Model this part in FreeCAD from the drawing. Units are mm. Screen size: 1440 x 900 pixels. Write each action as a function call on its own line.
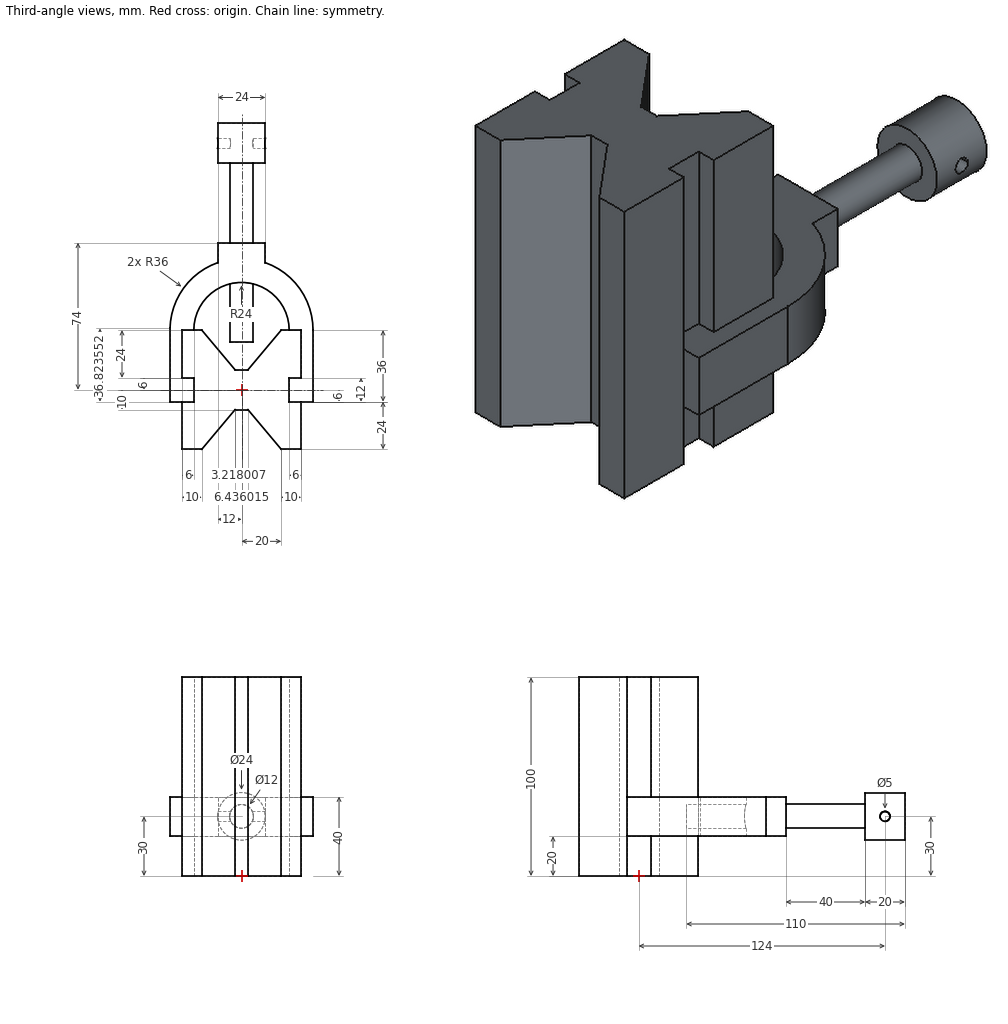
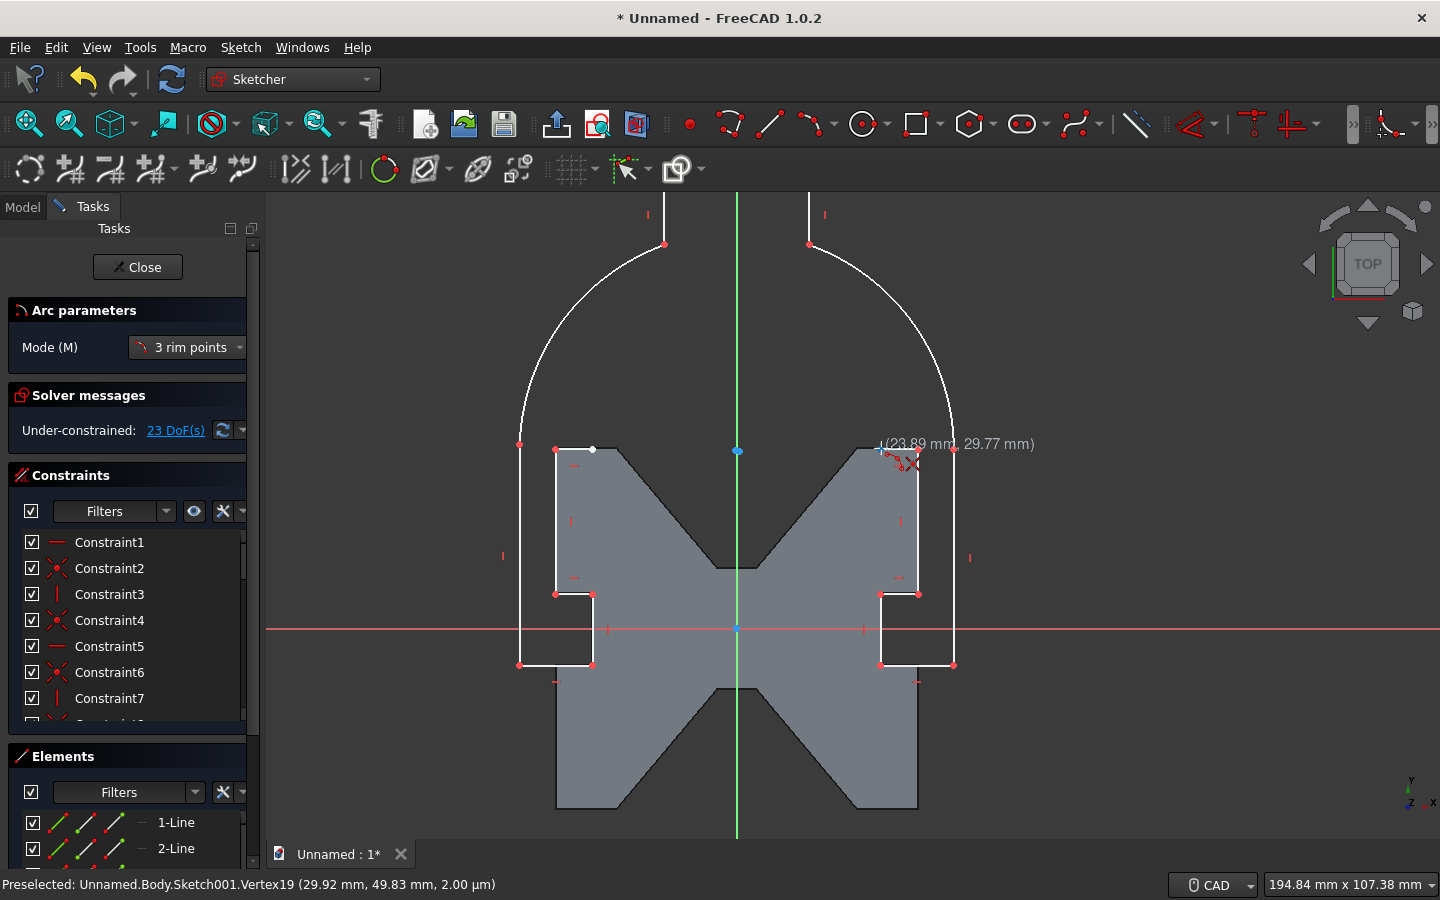
click(881, 449)
click(593, 449)
click(781, 310)
key(Escape)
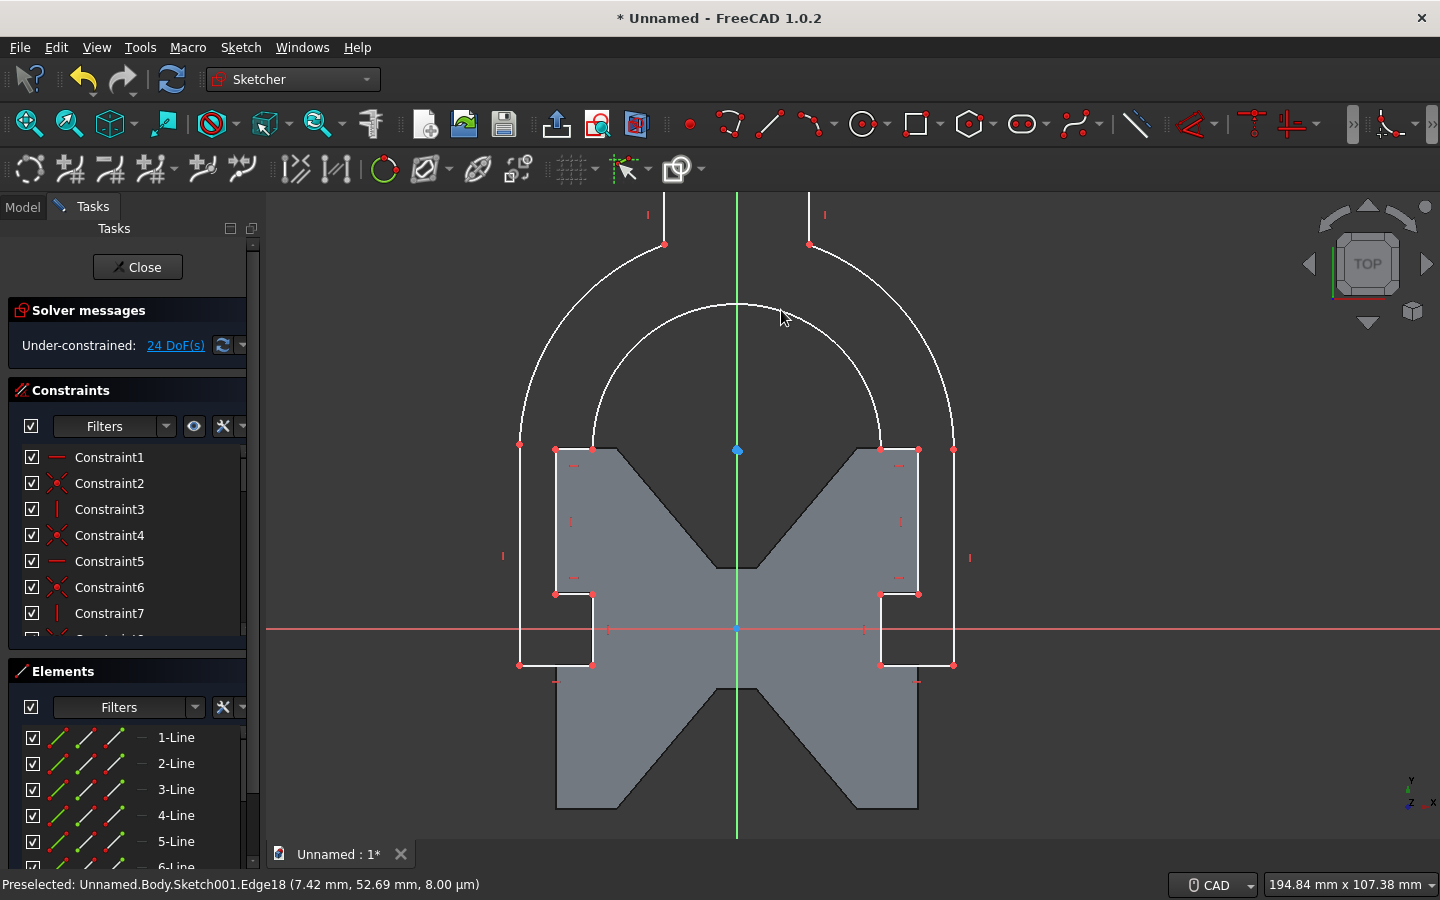
click(954, 514)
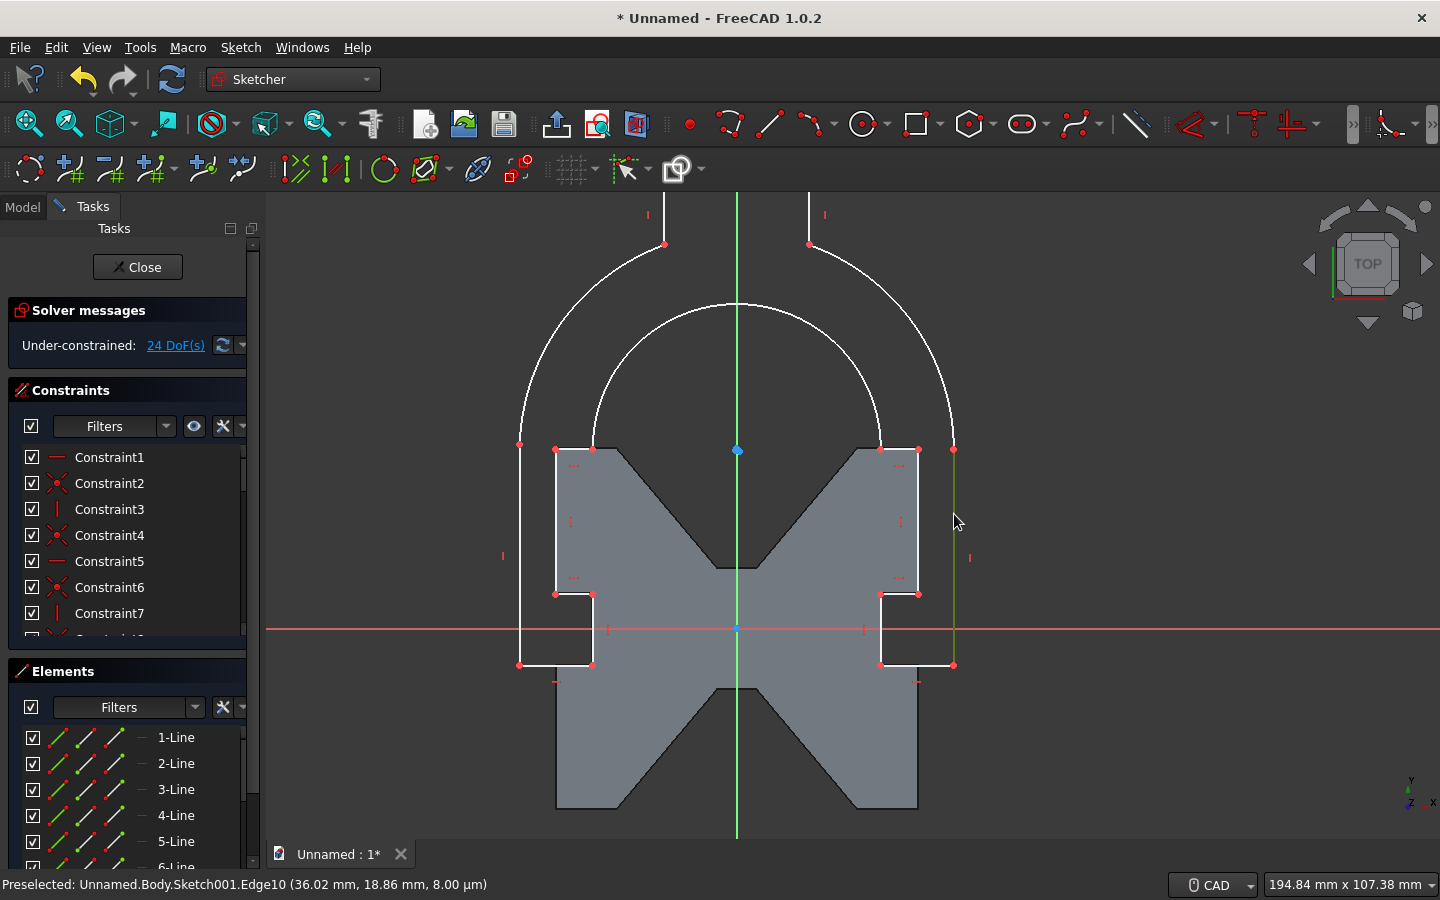
click(939, 371)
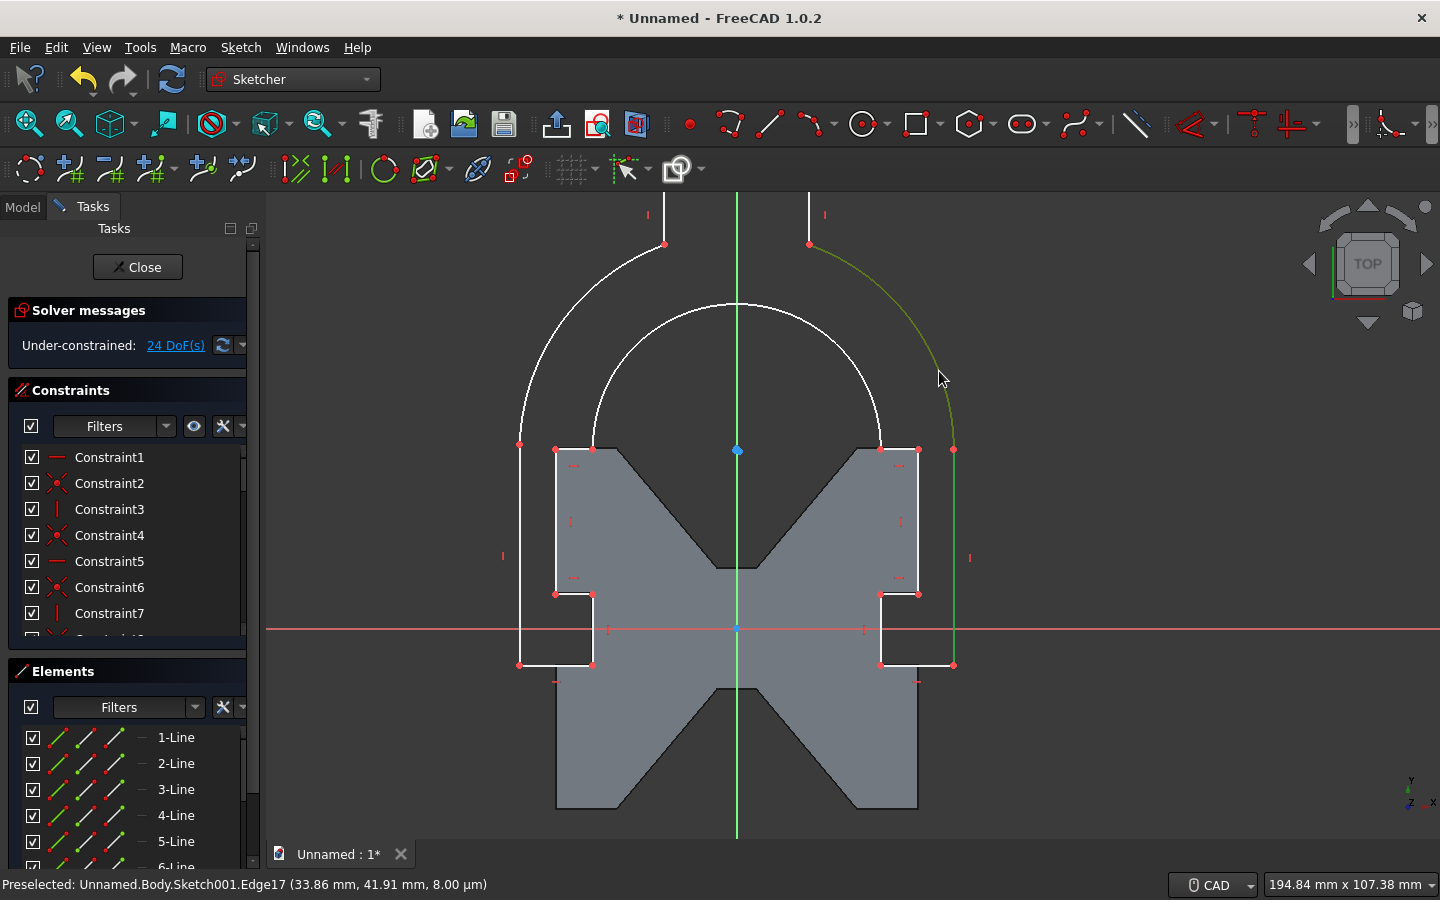
key(t)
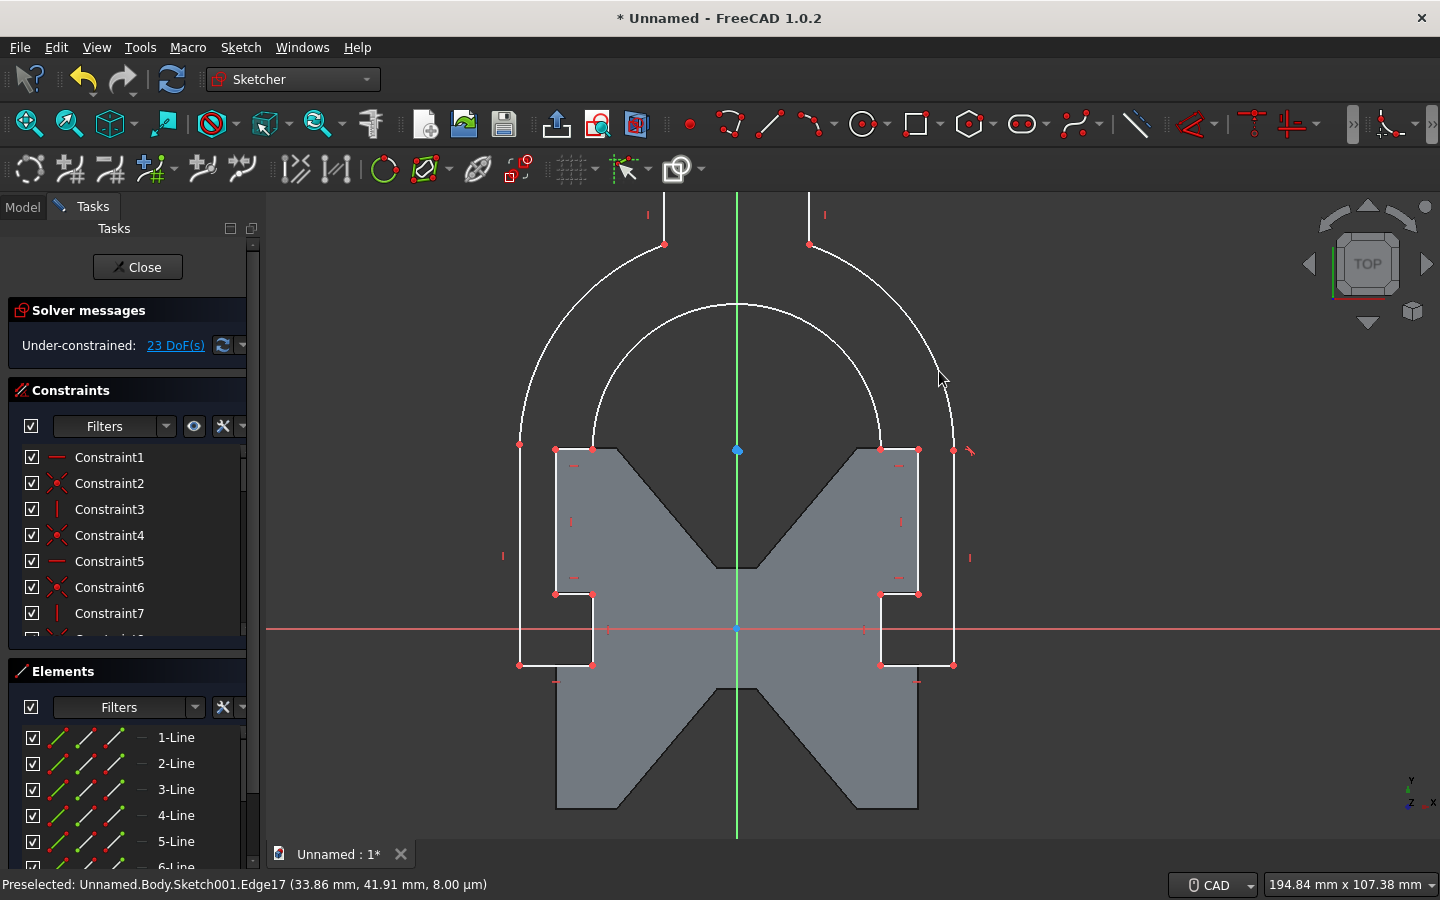
click(597, 284)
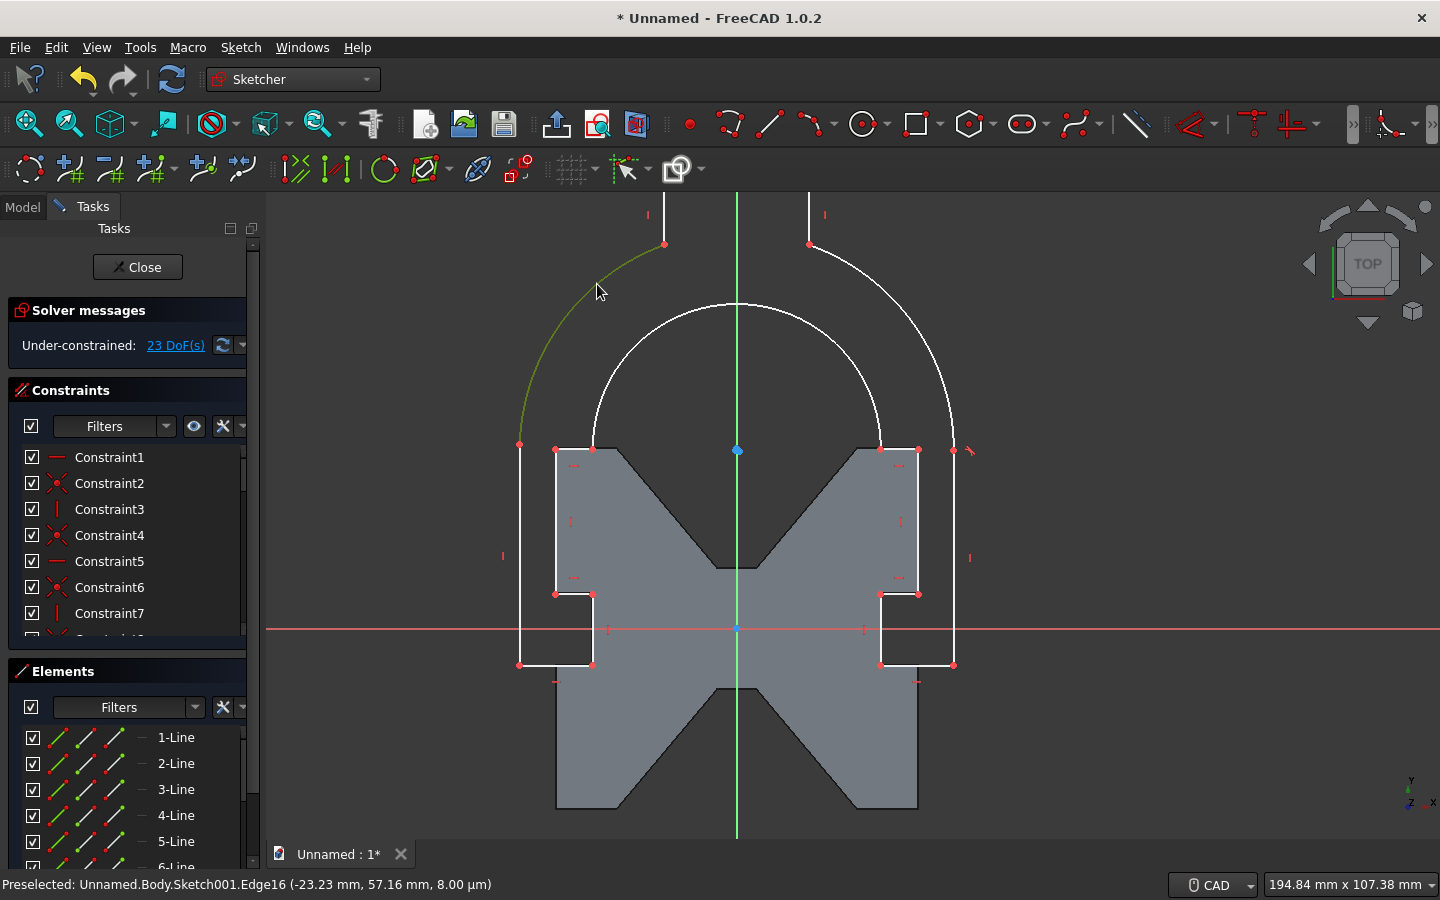
click(939, 372)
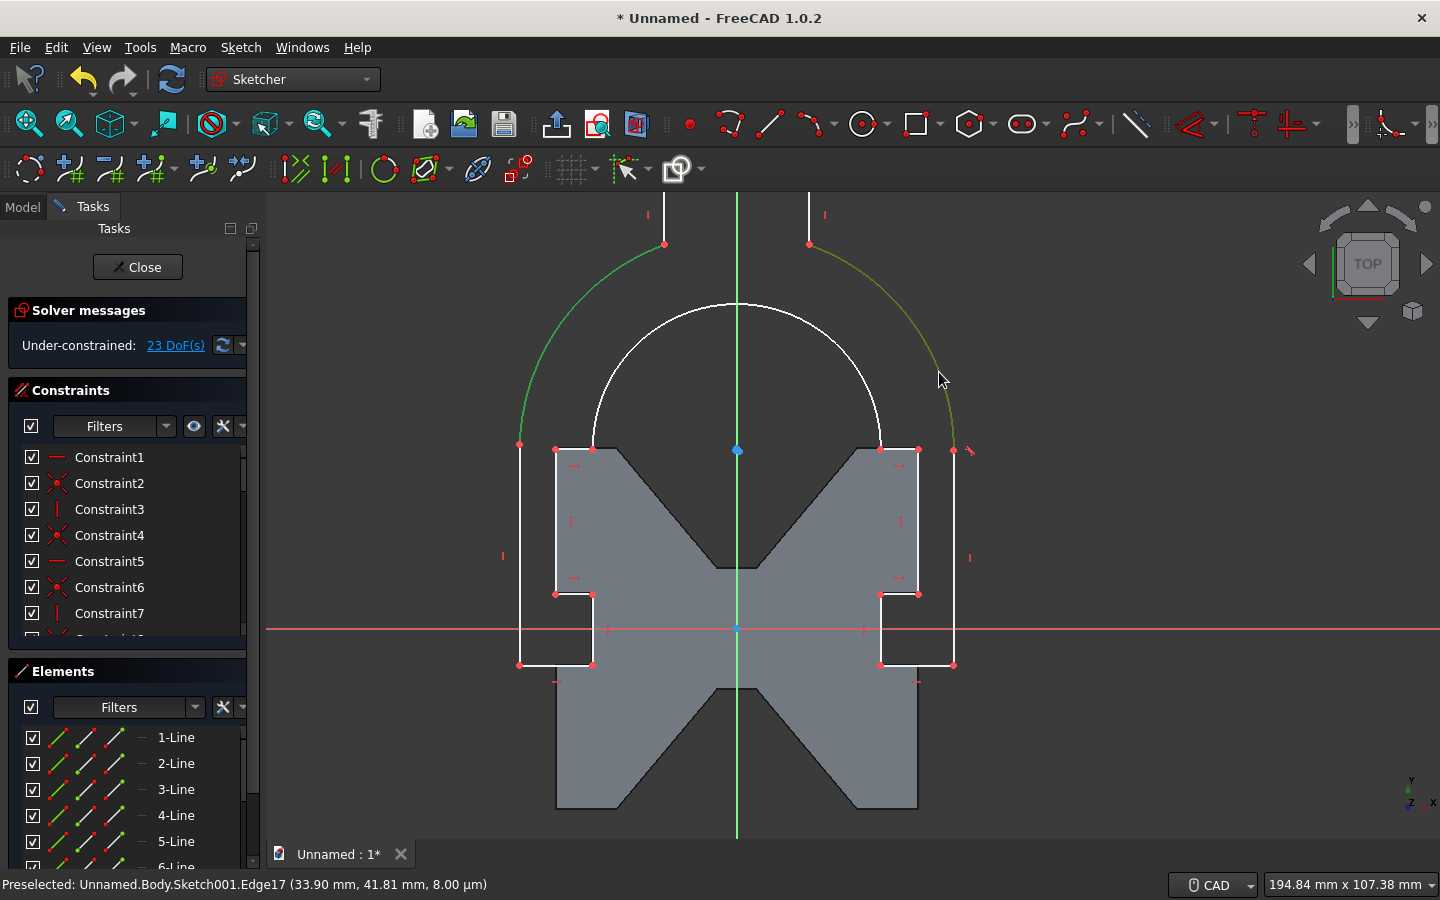
key(c)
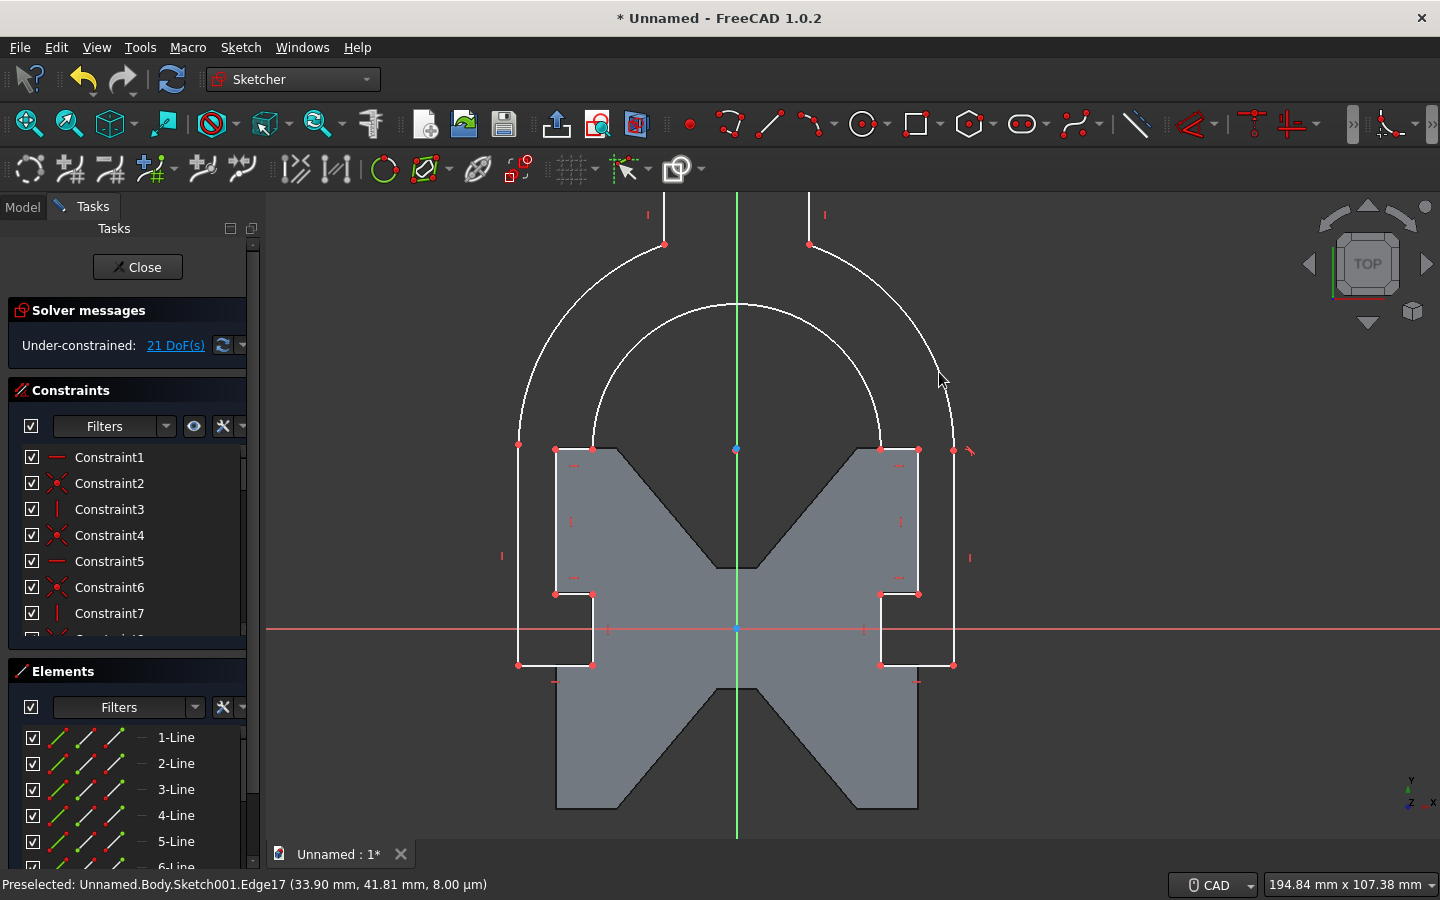
click(596, 284)